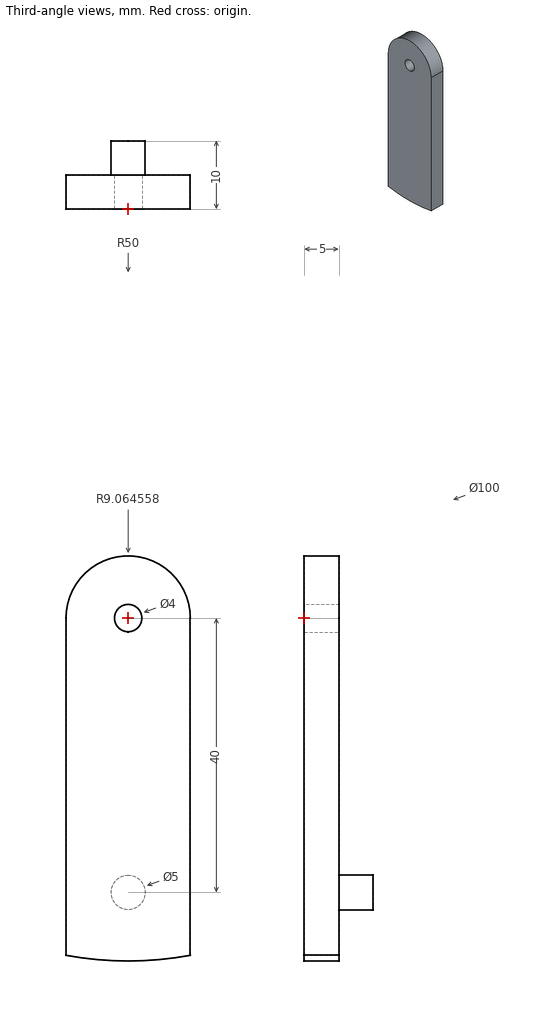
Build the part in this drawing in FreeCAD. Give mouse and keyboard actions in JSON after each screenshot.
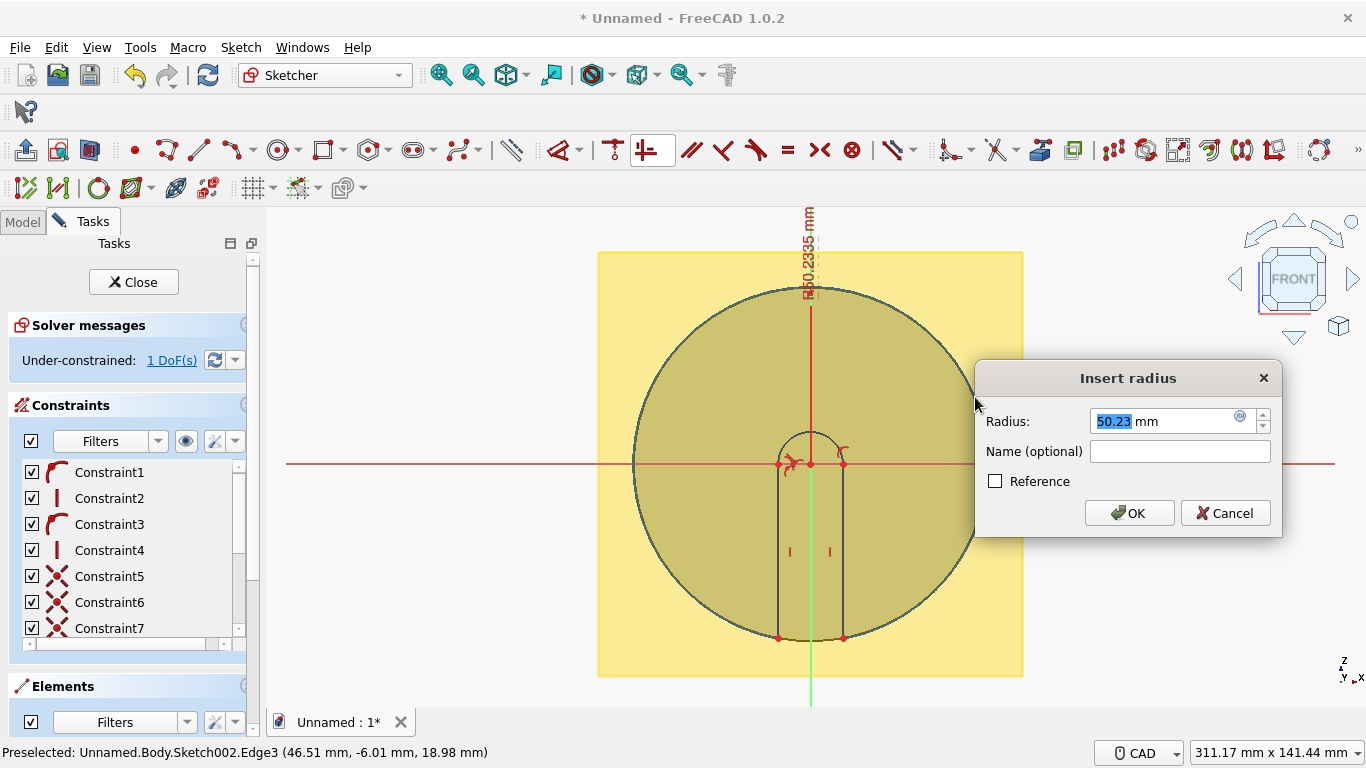
{"action": "type", "text": "50"}
{"action": "key", "text": "Return"}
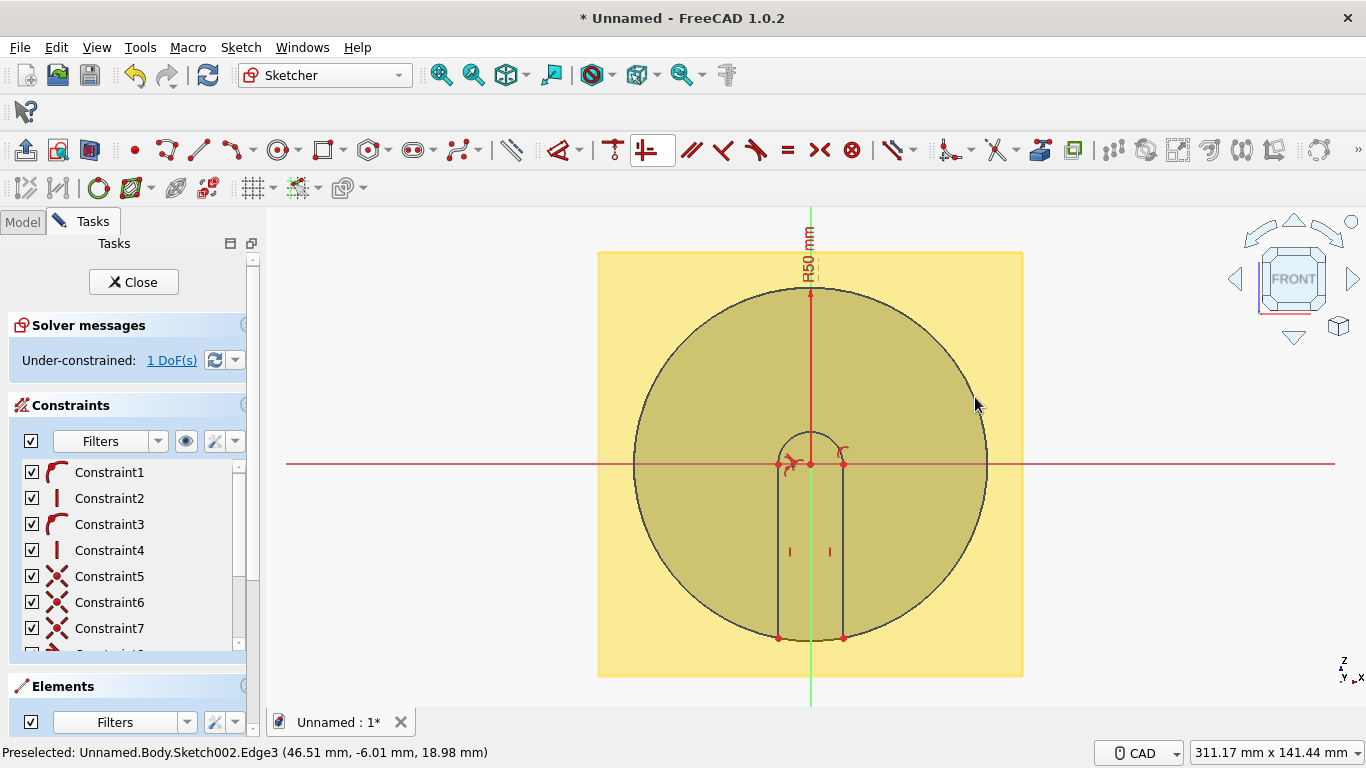
{"action": "scroll", "coordinate": [830, 438], "scroll_direction": "up", "scroll_amount": 2}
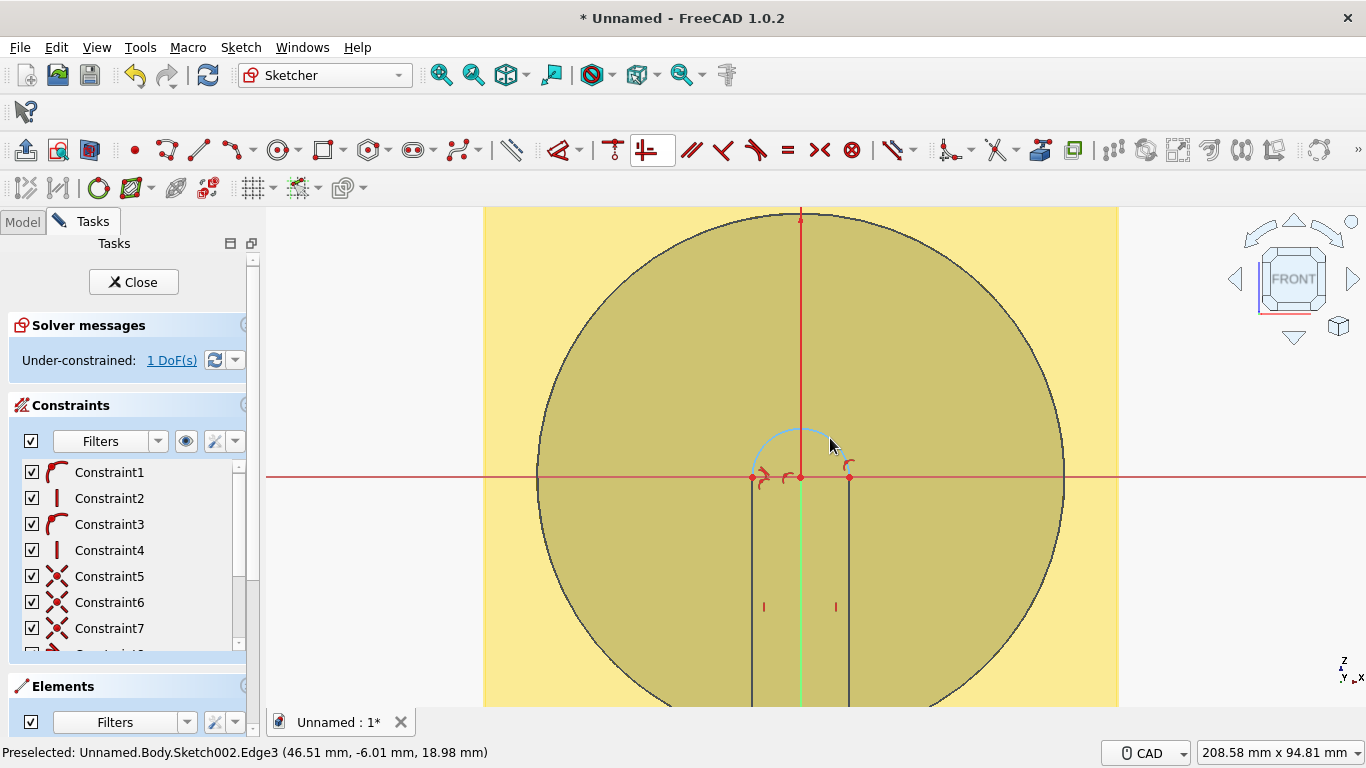
{"action": "left_click", "coordinate": [829, 438]}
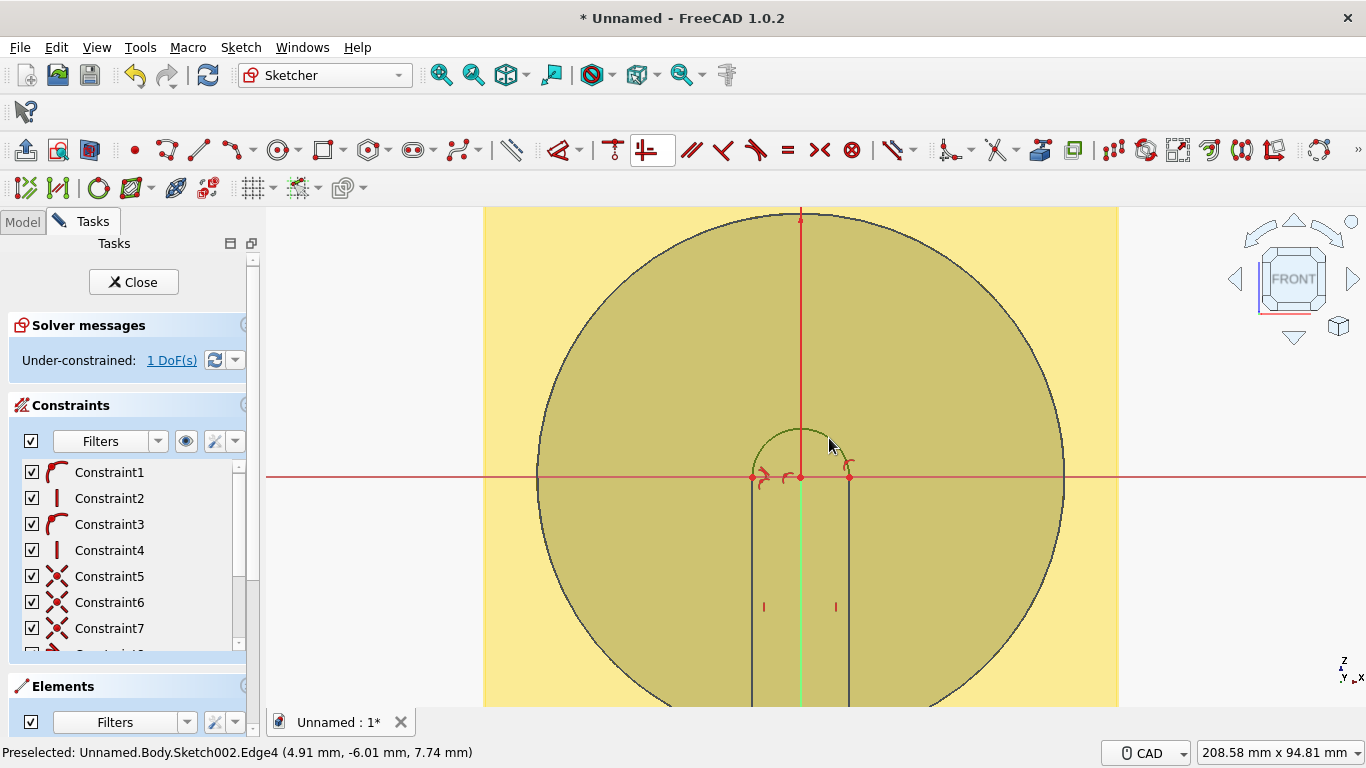
{"action": "key", "text": "k r"}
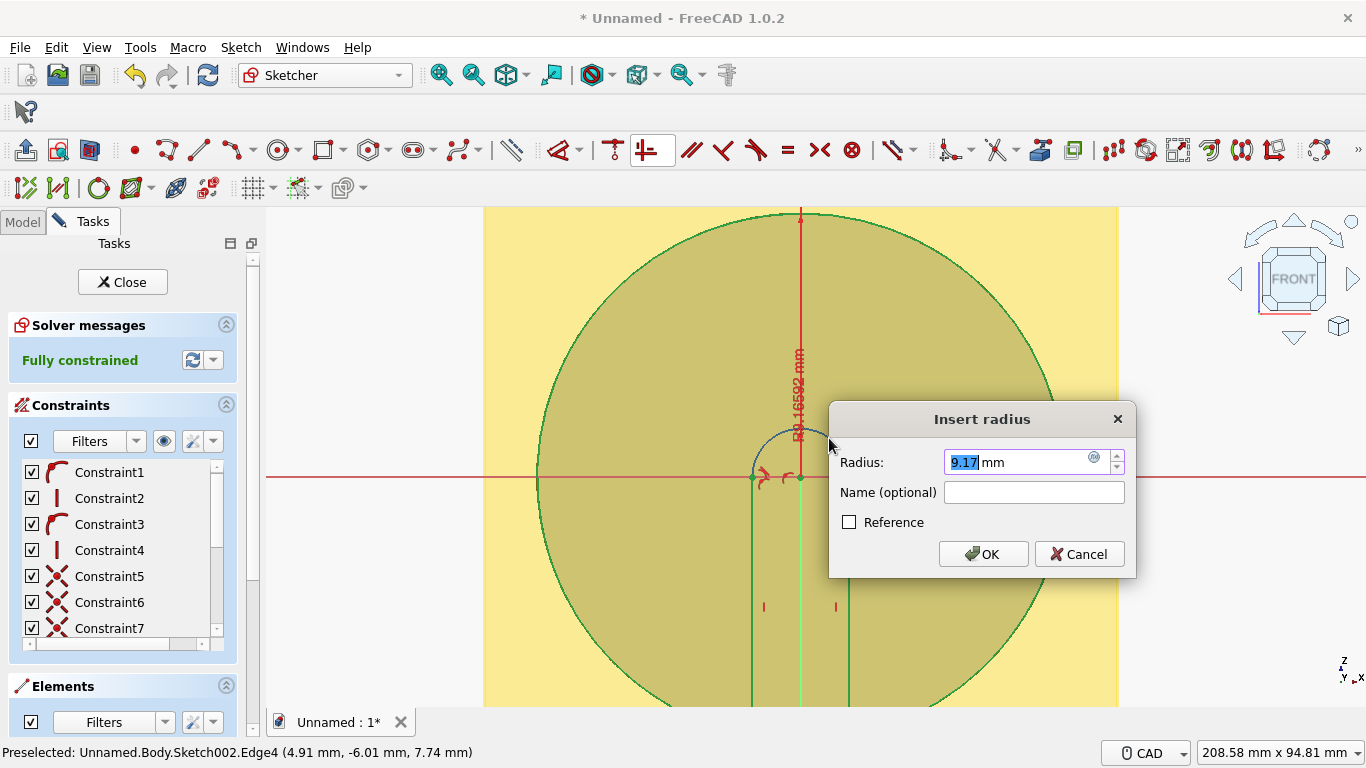
{"action": "type", "text": "9.064558"}
{"action": "key", "text": "Return"}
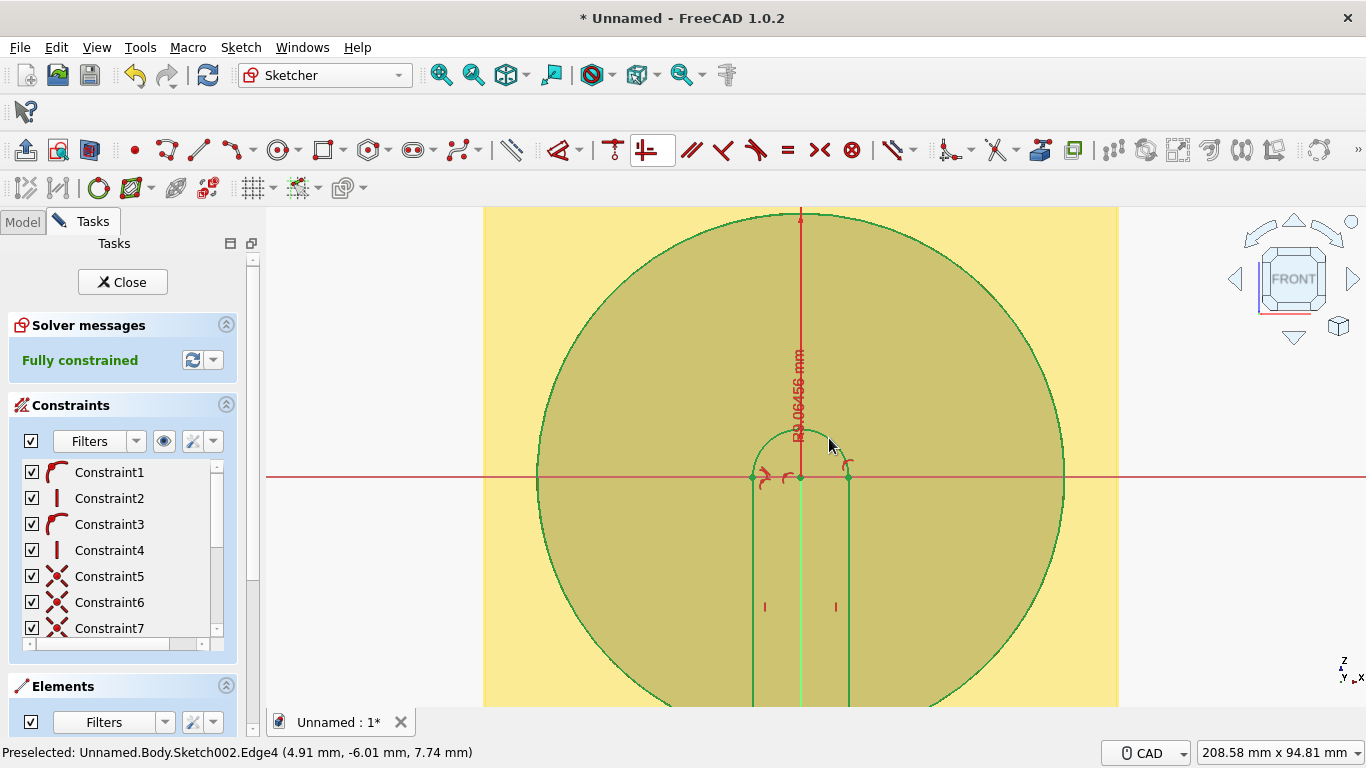
{"action": "left_click", "coordinate": [123, 282]}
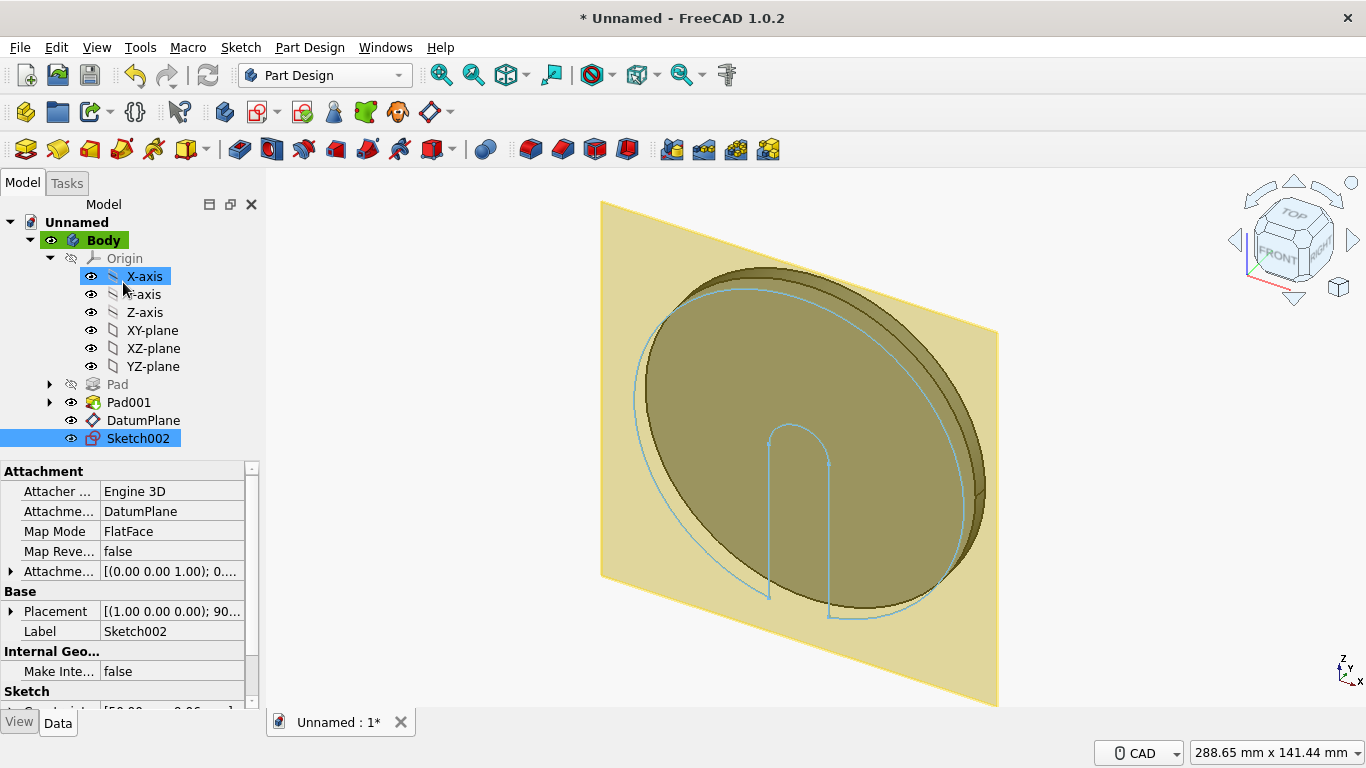
{"action": "left_click", "coordinate": [240, 150]}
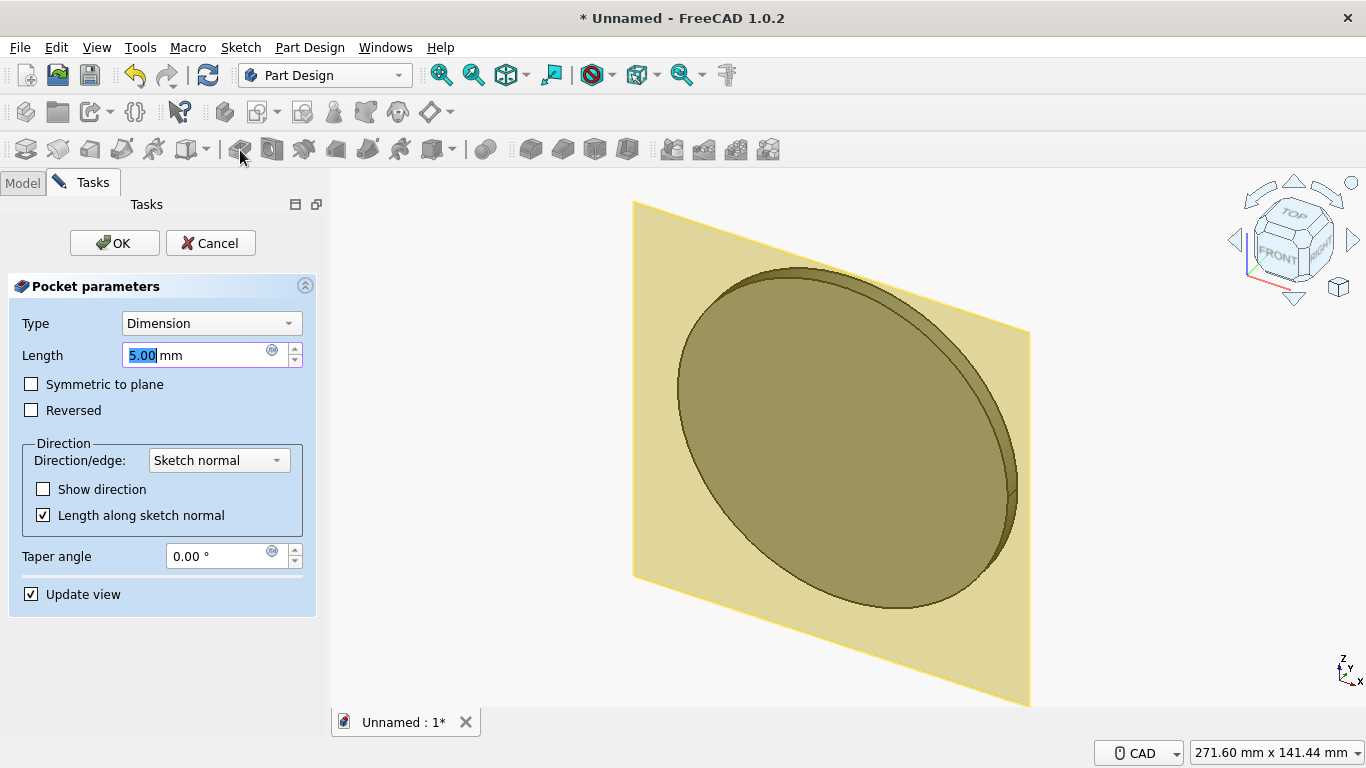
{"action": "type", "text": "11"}
{"action": "key", "text": "Tab"}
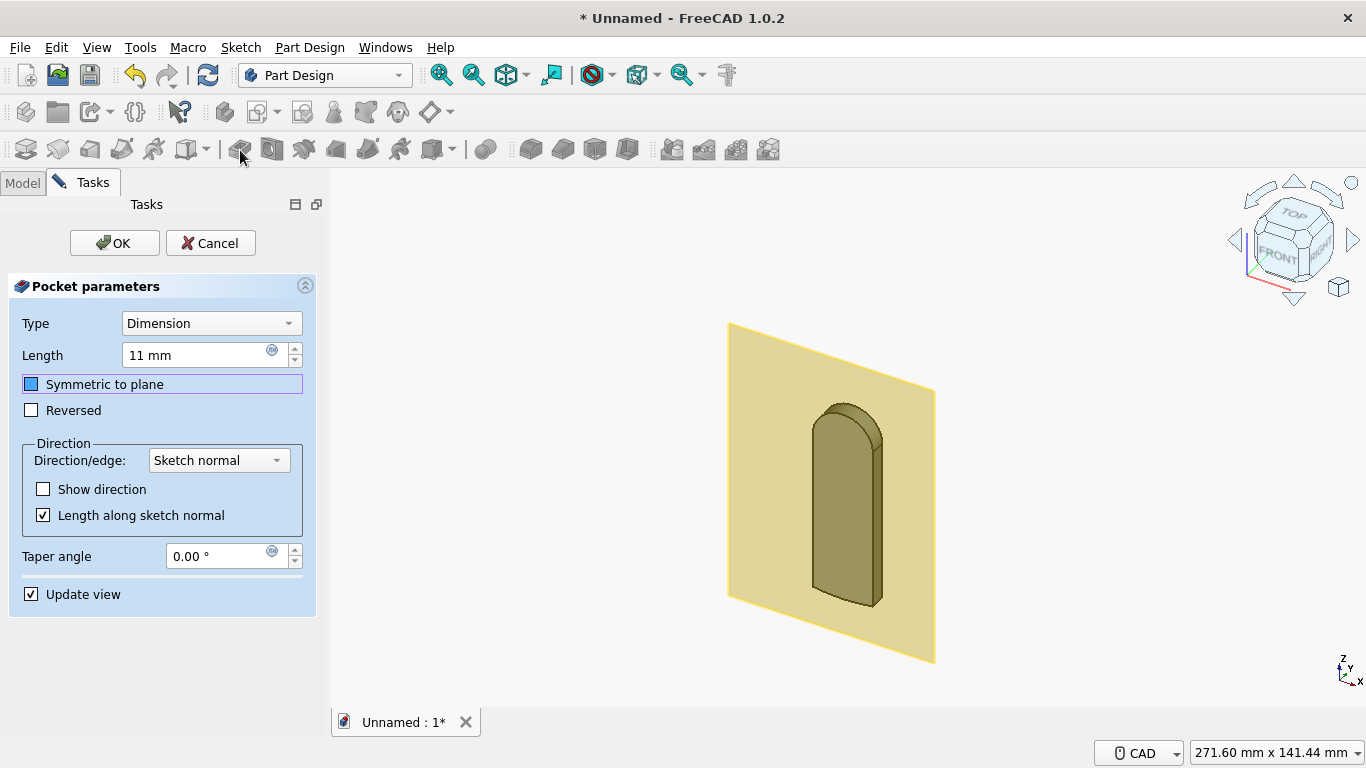
{"action": "left_click", "coordinate": [115, 243]}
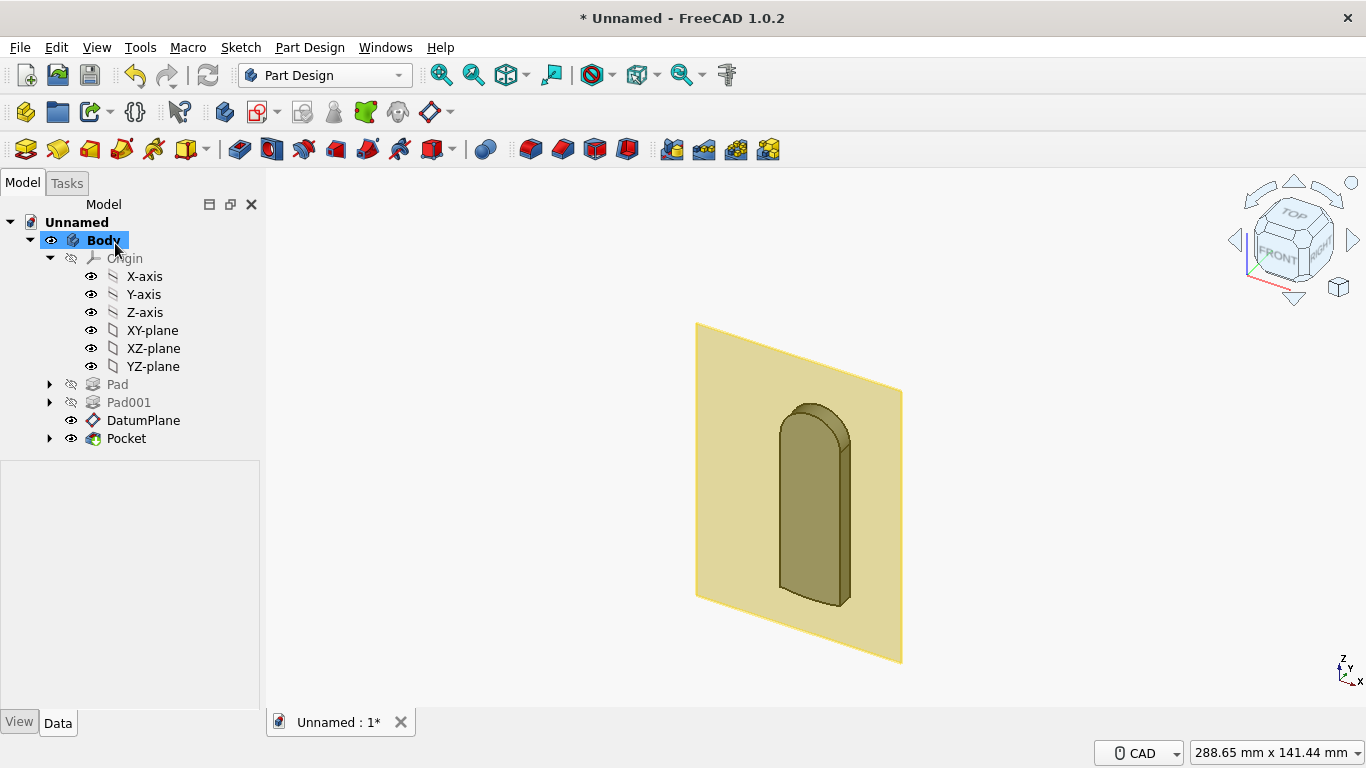
{"action": "left_click", "coordinate": [116, 420]}
{"action": "key", "text": "space"}